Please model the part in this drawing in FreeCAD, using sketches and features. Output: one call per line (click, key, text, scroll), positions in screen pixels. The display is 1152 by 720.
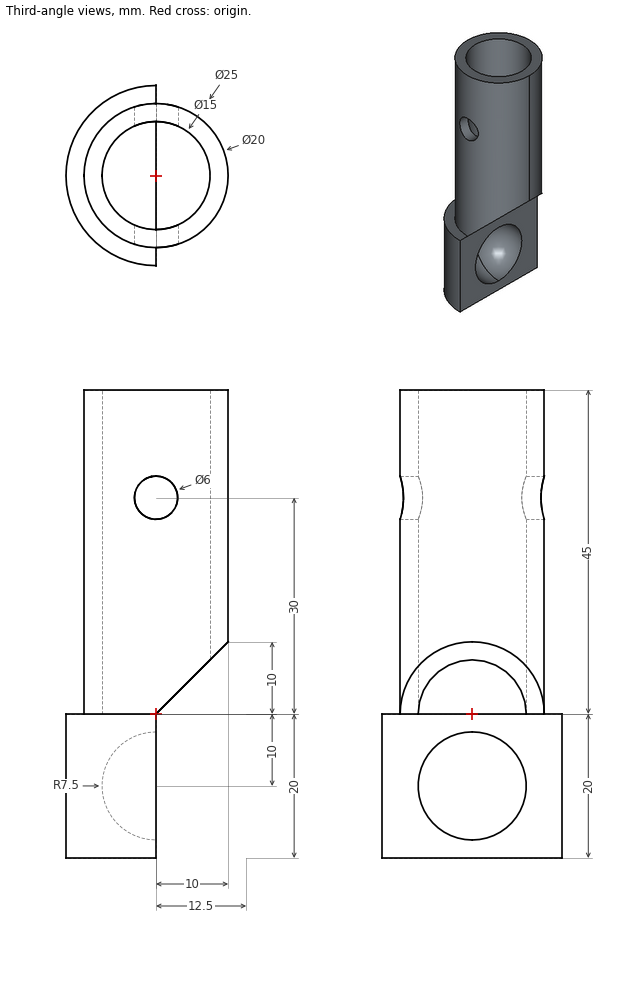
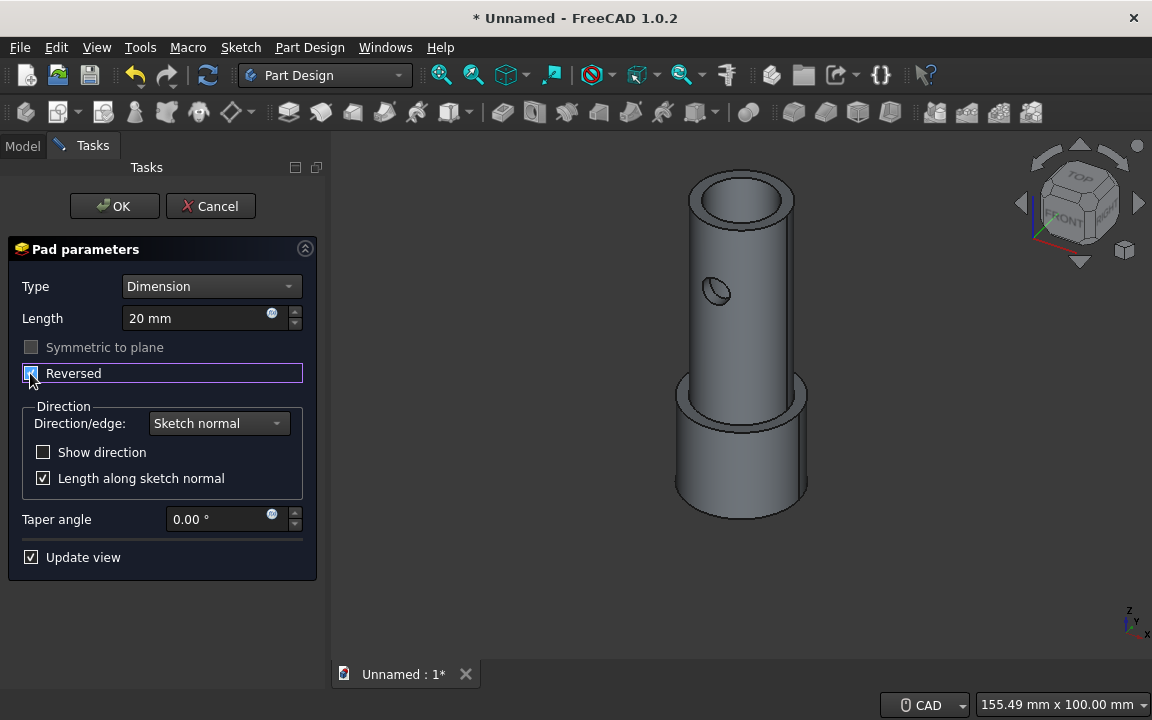
click(115, 206)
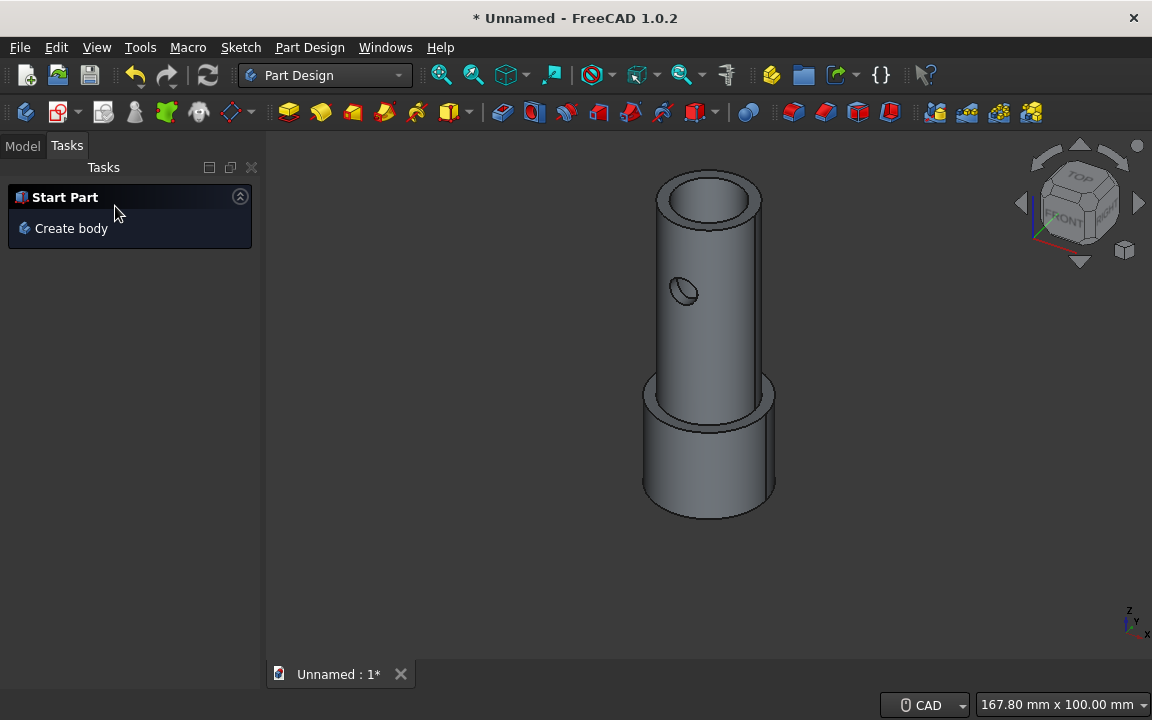
click(58, 112)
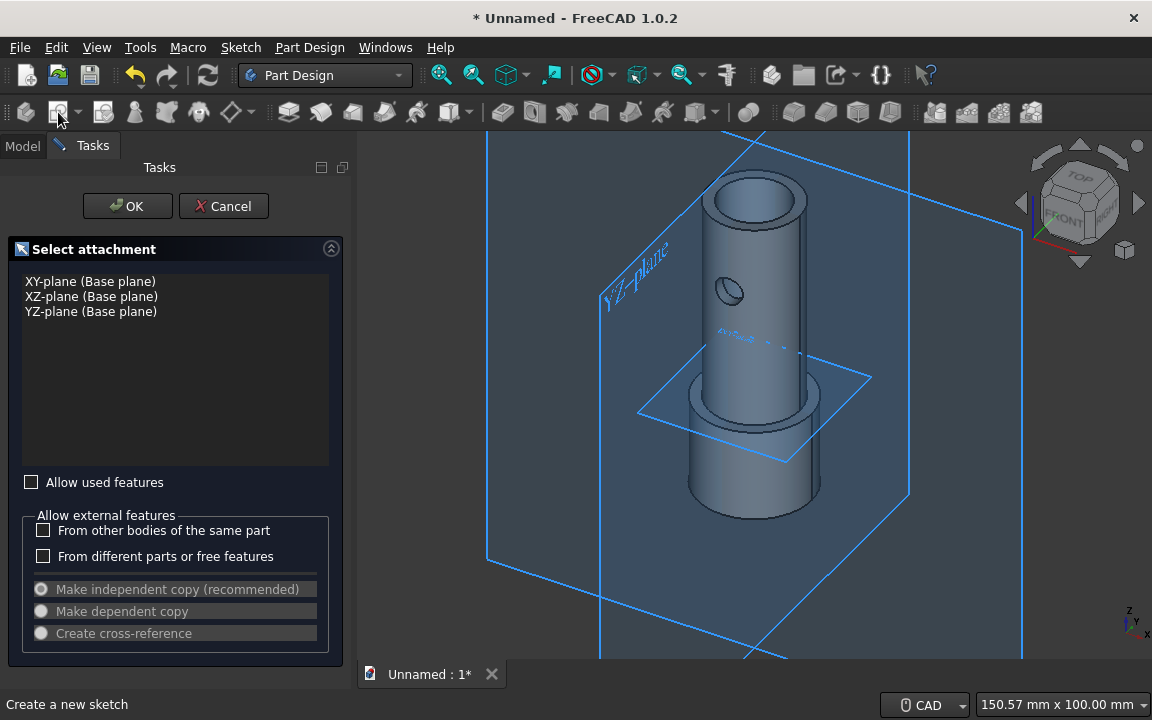
click(82, 296)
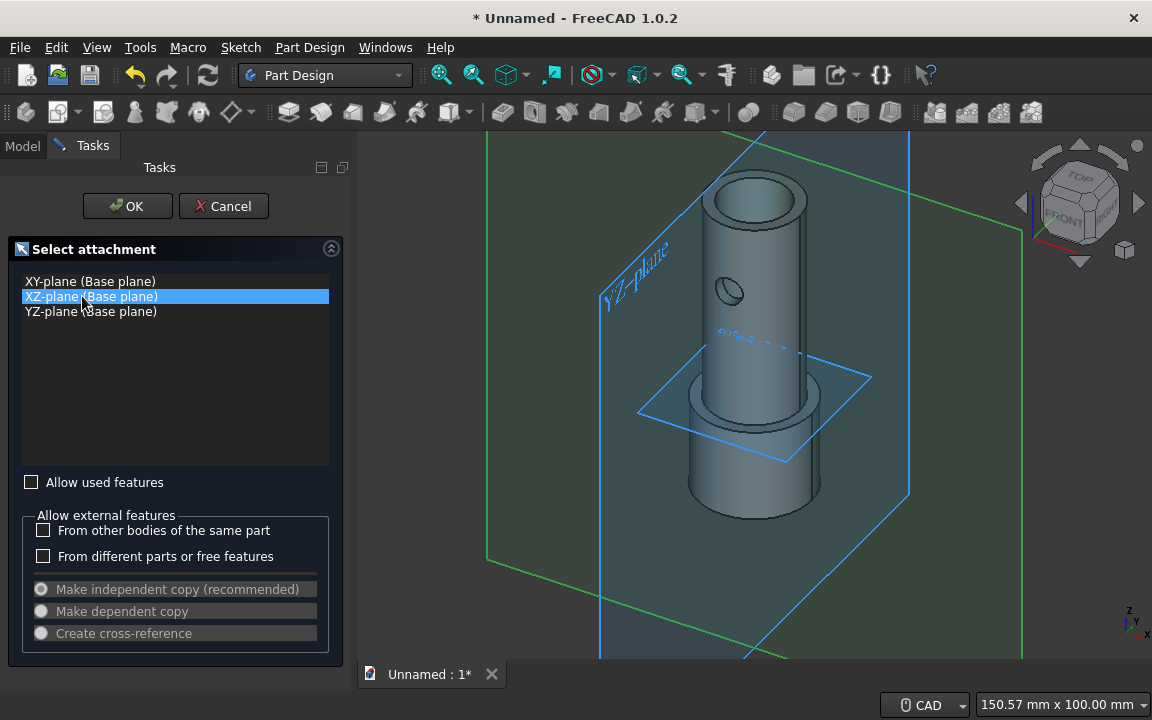
click(128, 206)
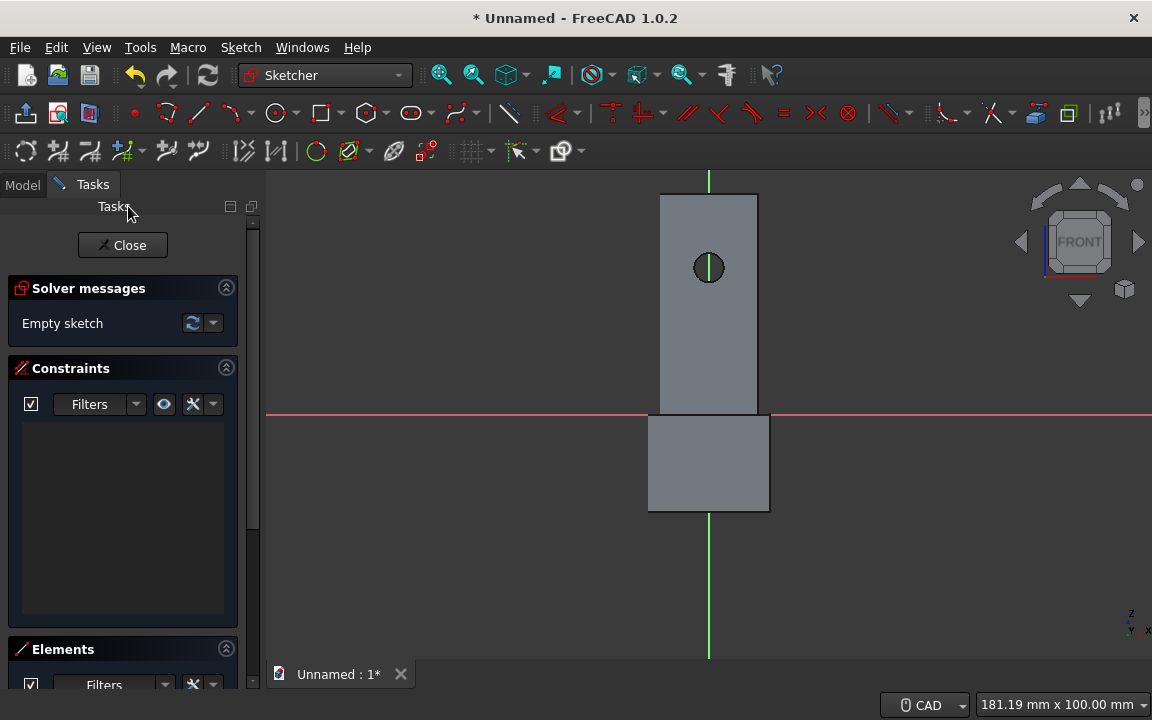
click(90, 114)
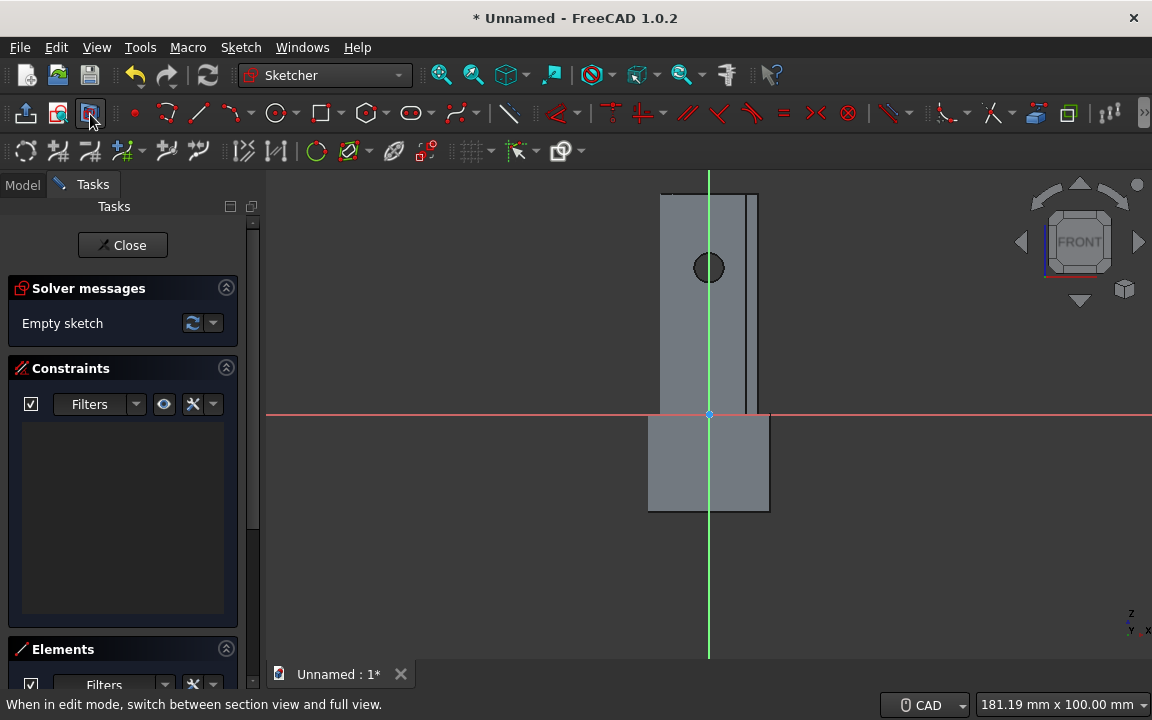
scroll(820, 459, up, 4)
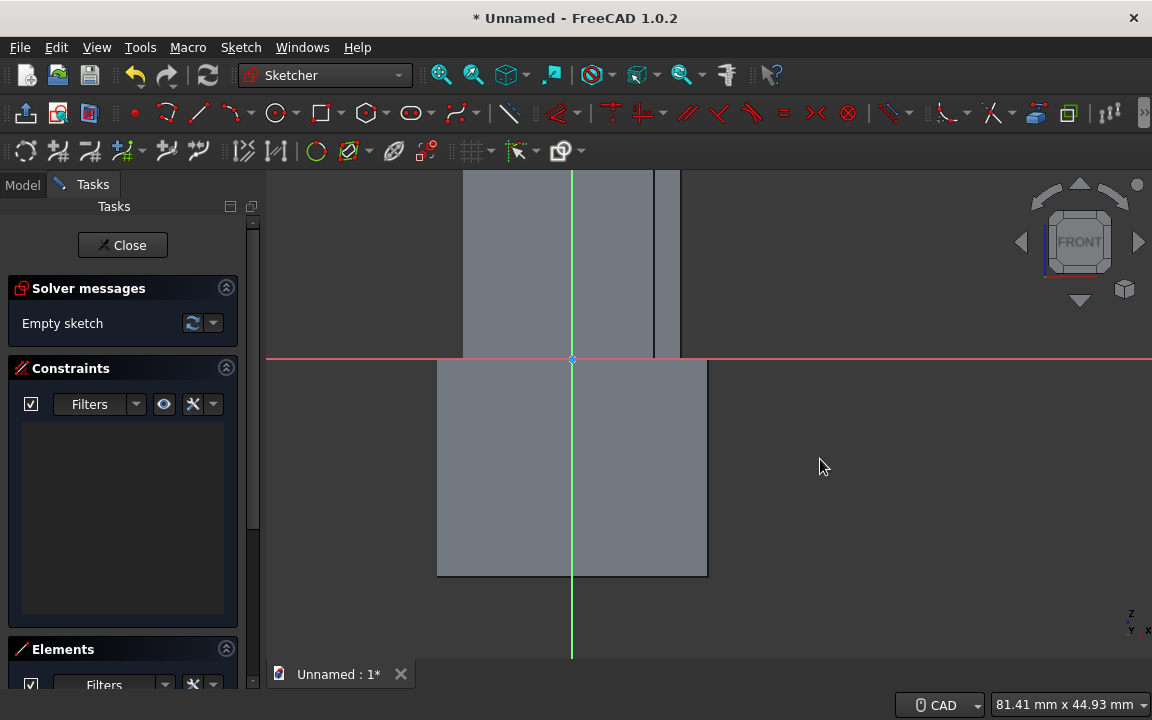
click(168, 114)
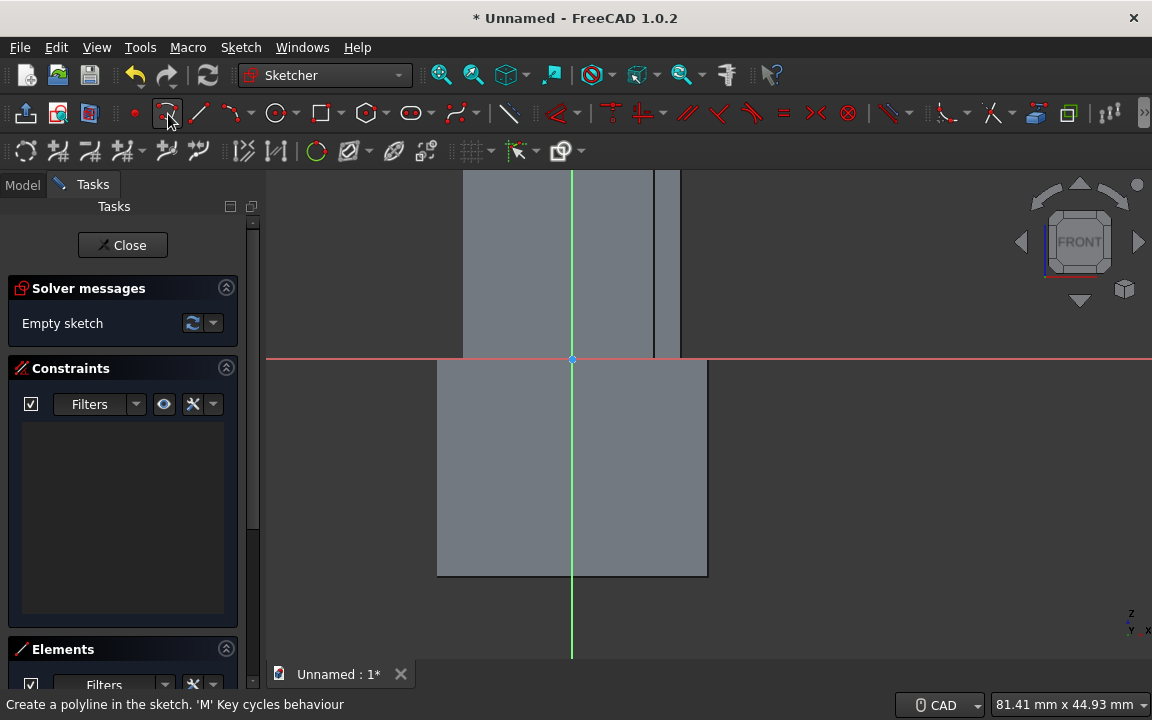
click(572, 359)
click(681, 250)
click(708, 359)
click(708, 577)
click(581, 577)
click(572, 359)
key(Escape)
key(Escape)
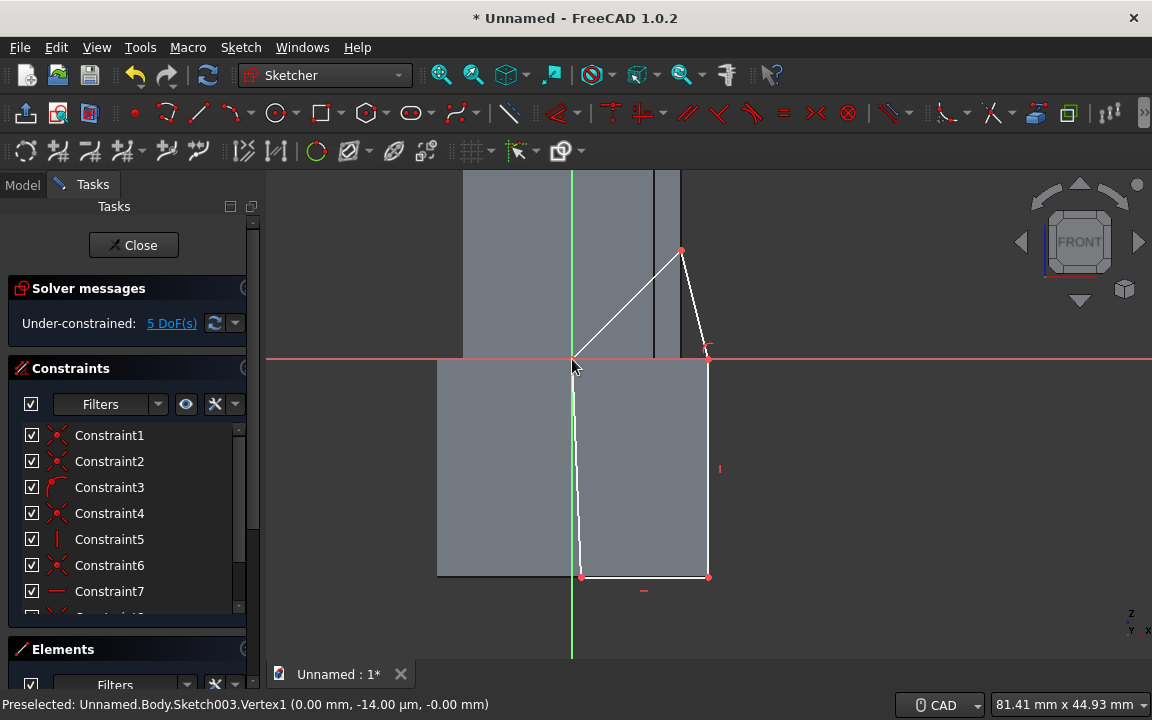
click(575, 425)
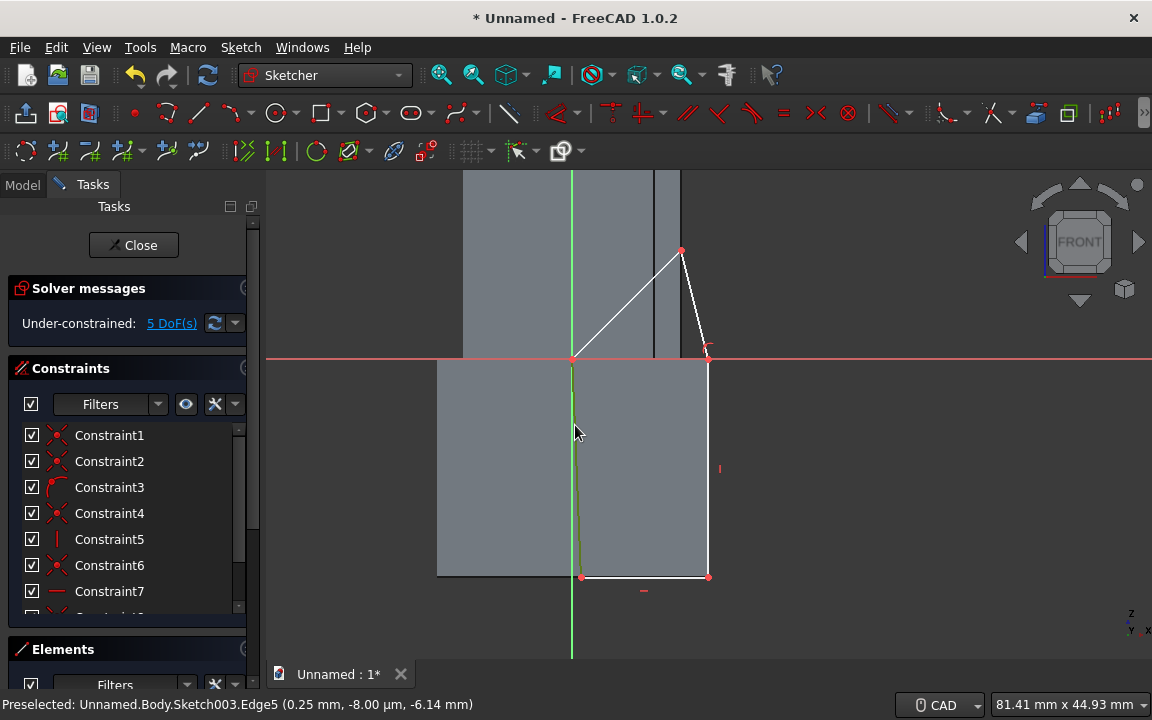
click(666, 114)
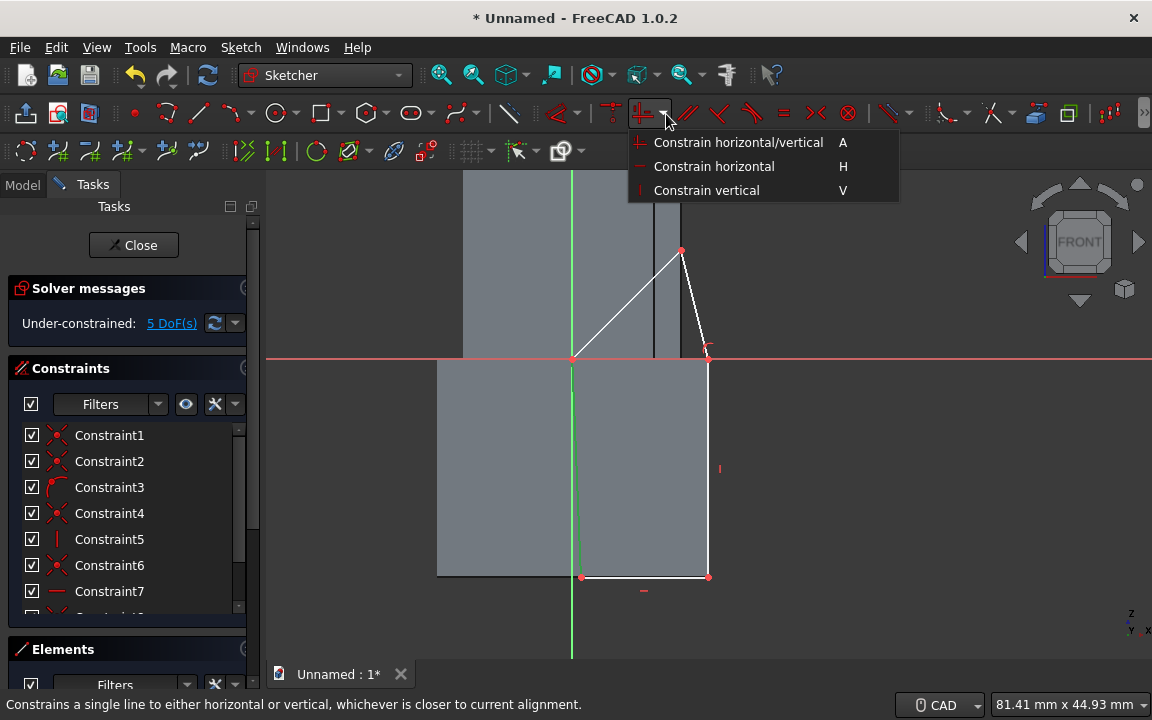
click(764, 190)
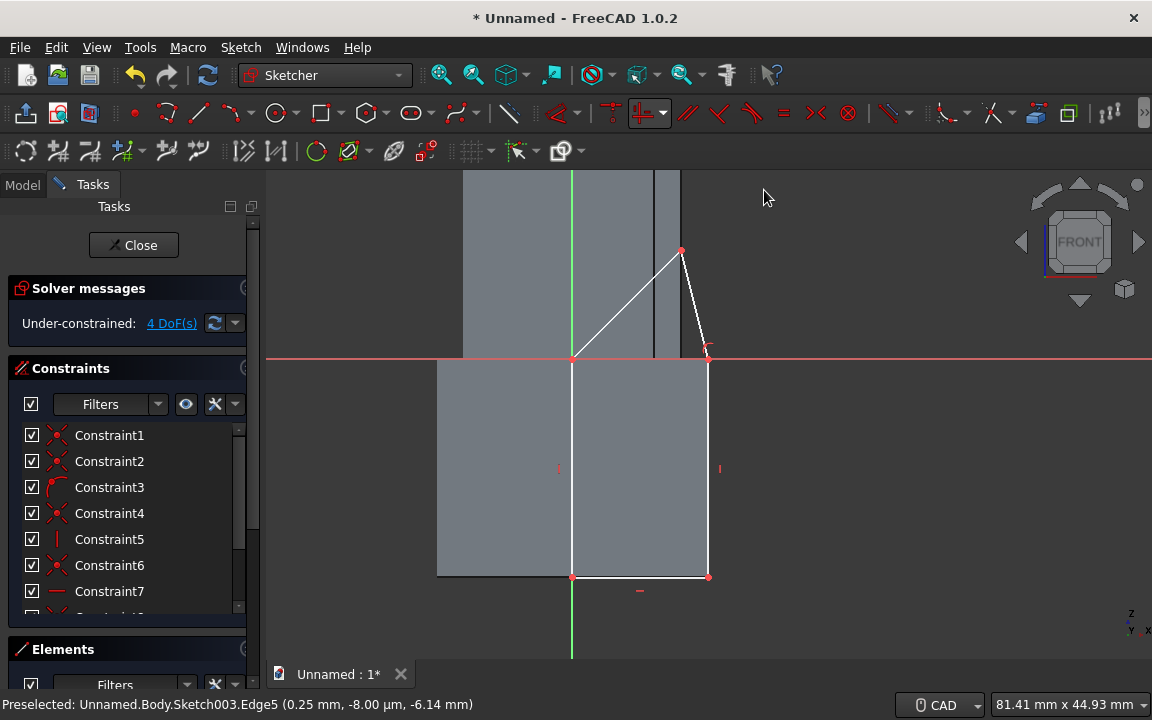
click(556, 114)